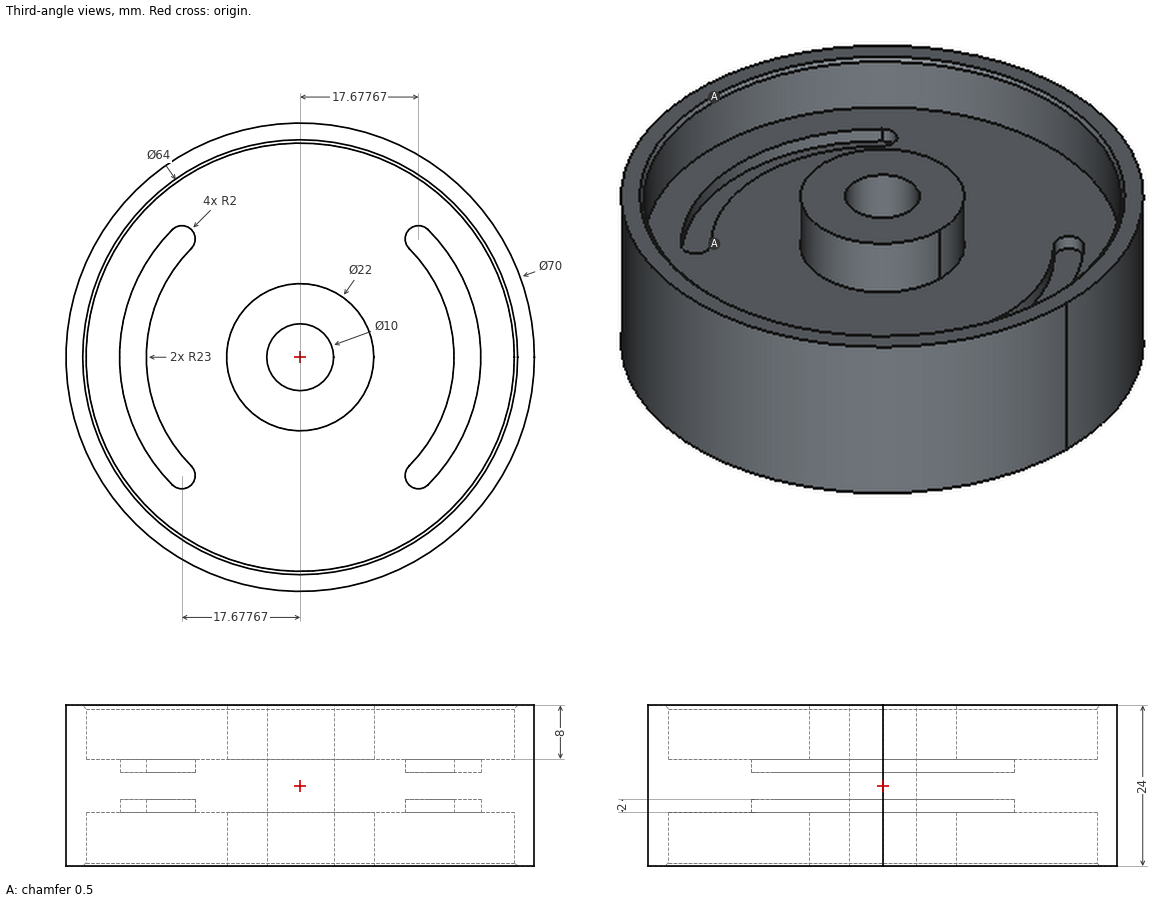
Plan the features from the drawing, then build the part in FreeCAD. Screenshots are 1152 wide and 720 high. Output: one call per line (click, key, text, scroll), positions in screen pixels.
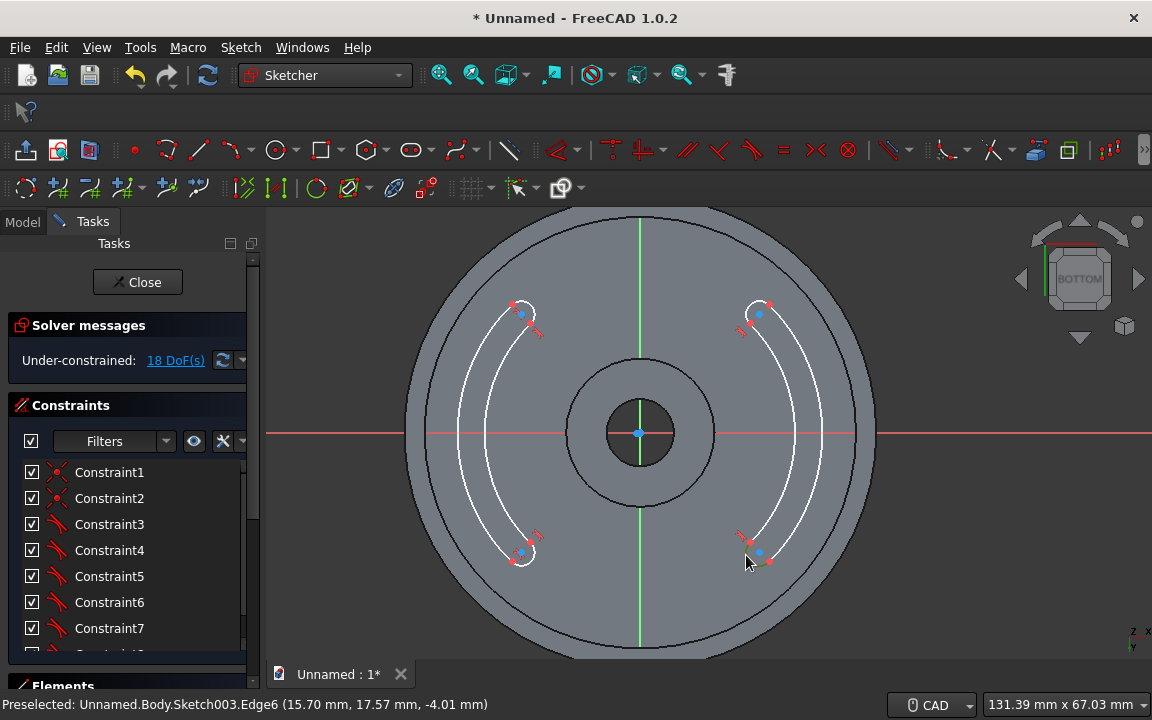
click(813, 490)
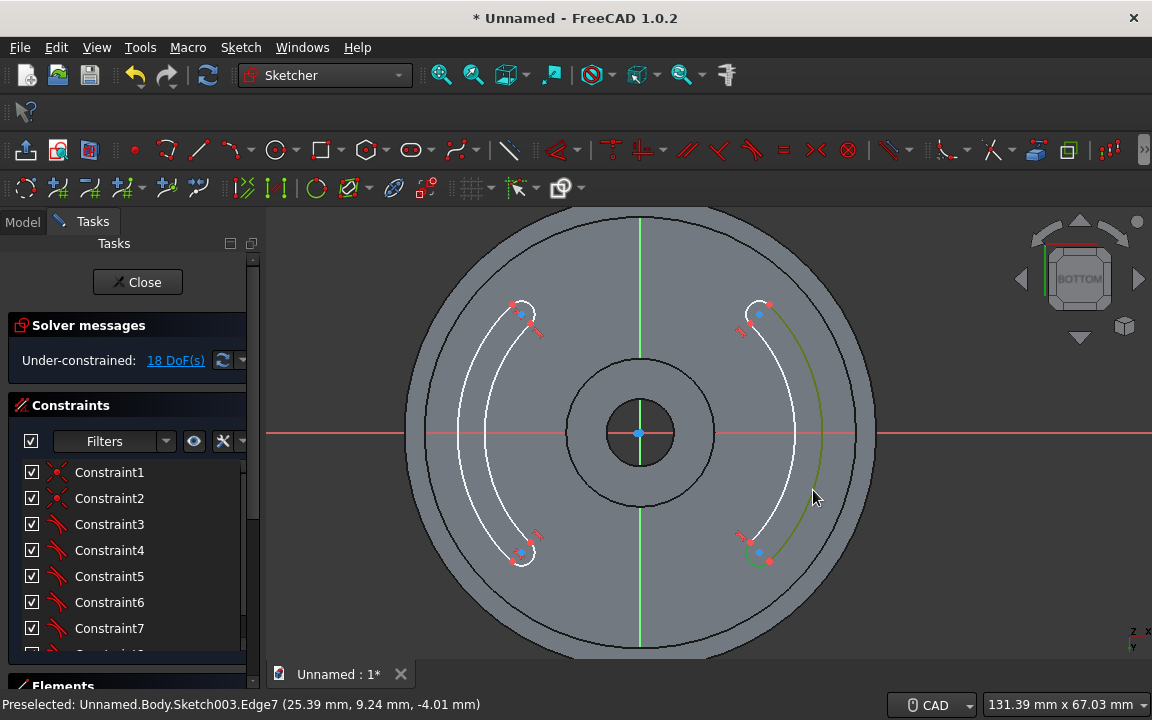
key(t)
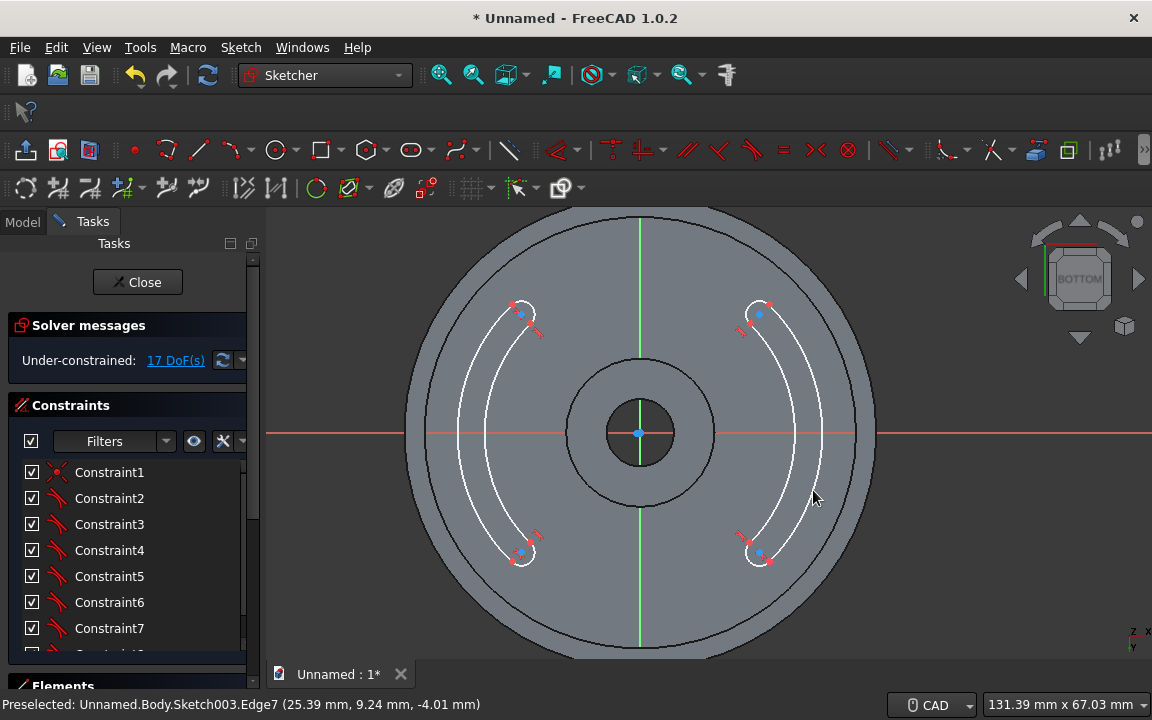
click(813, 490)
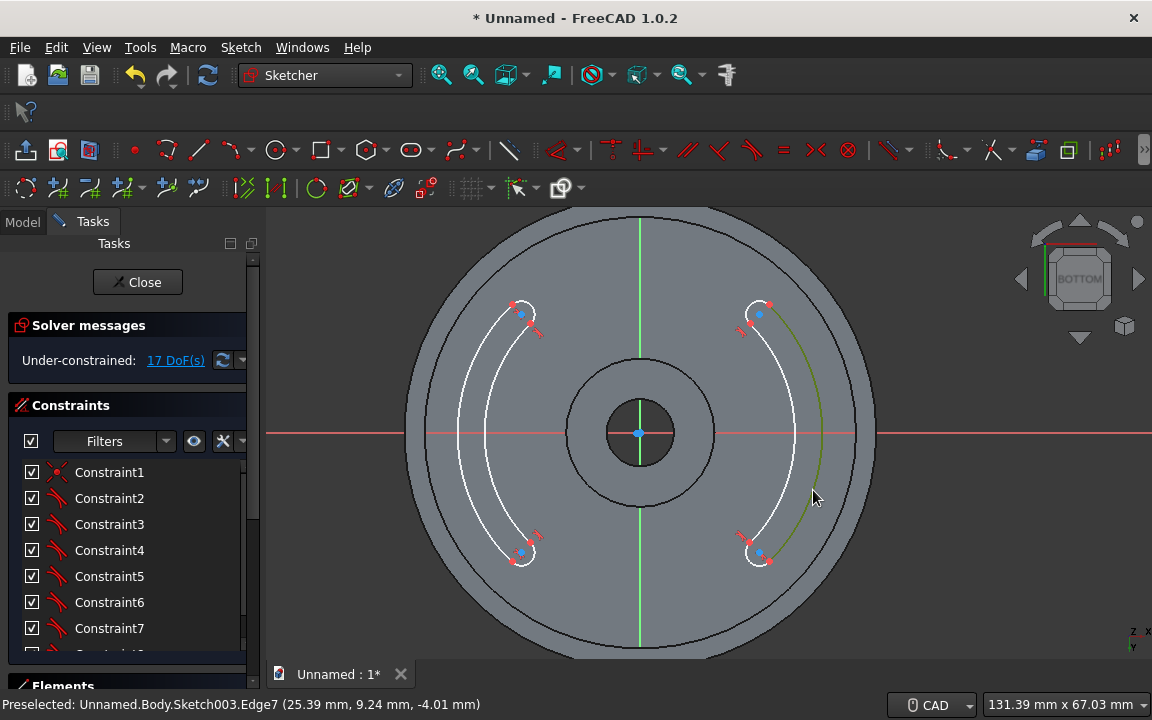
click(757, 301)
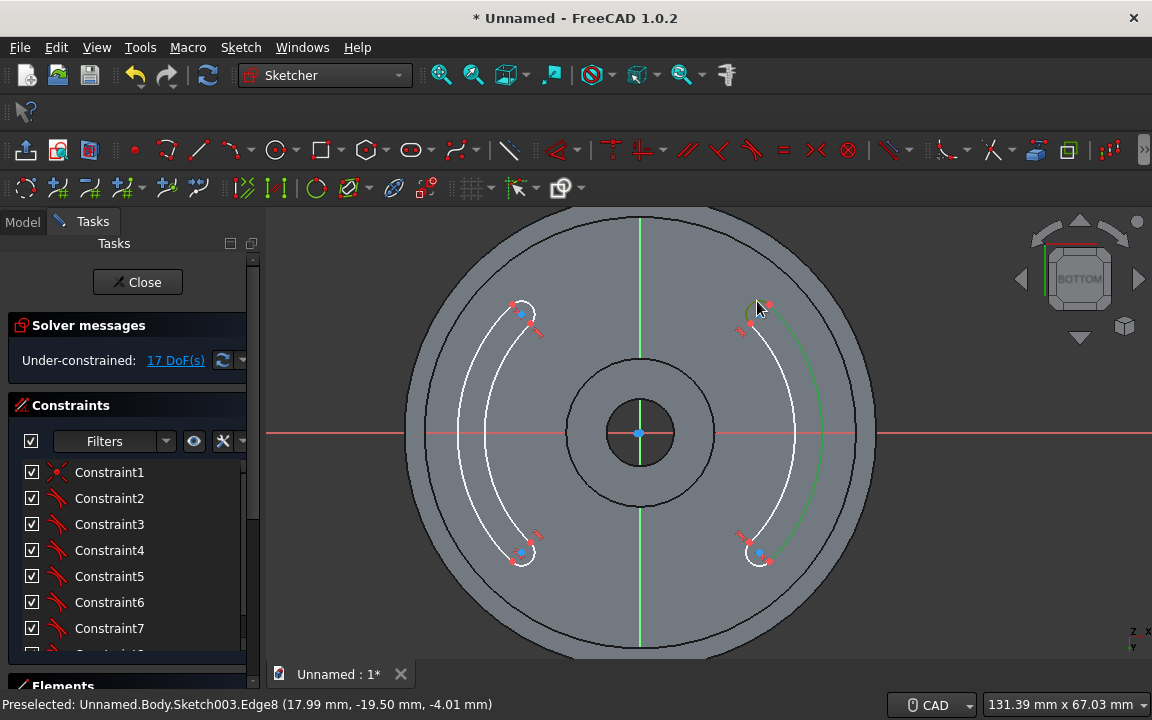
key(t)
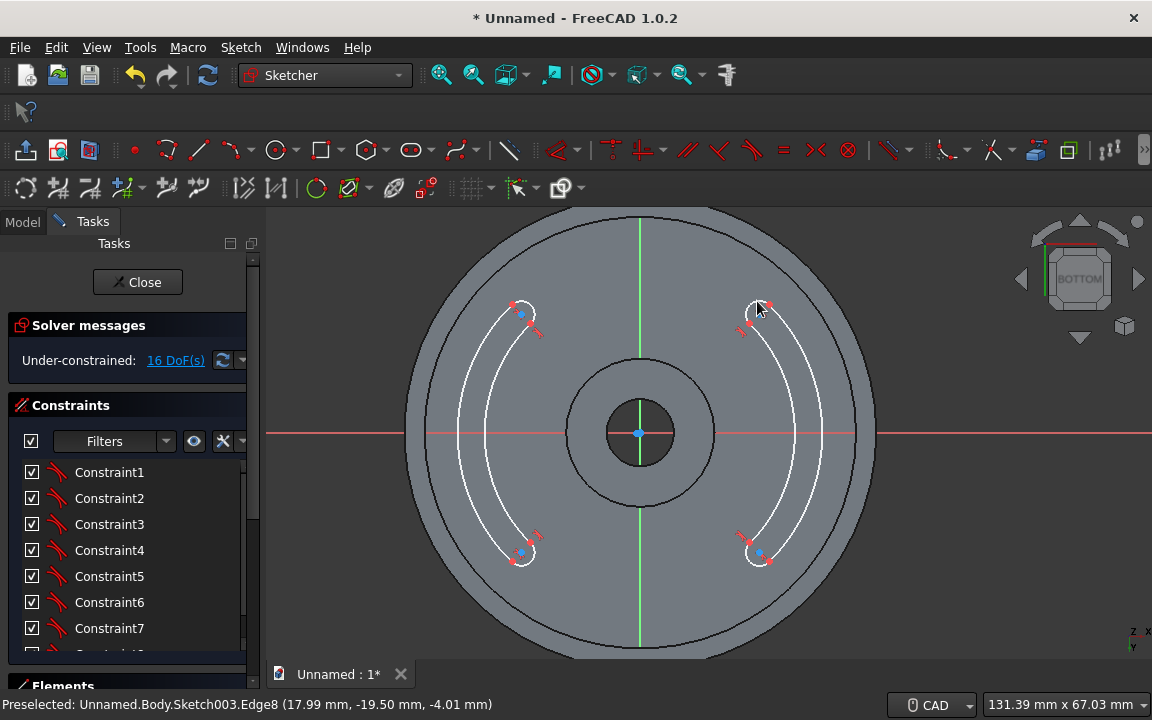
click(492, 386)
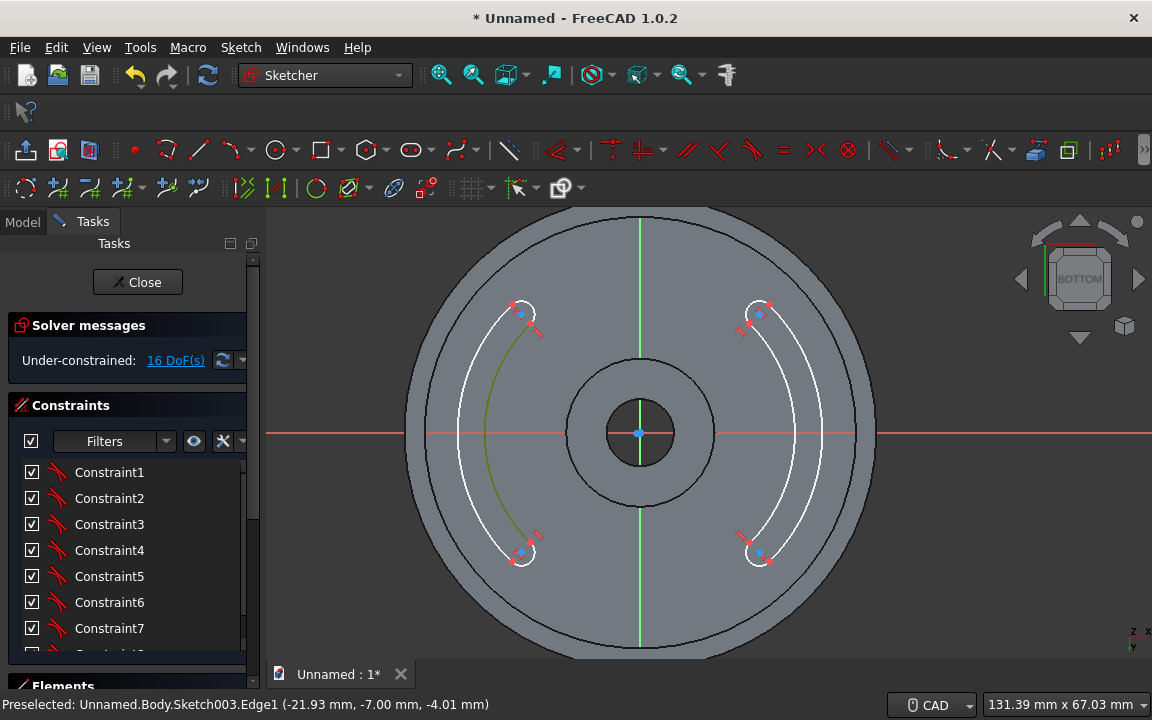
click(467, 377)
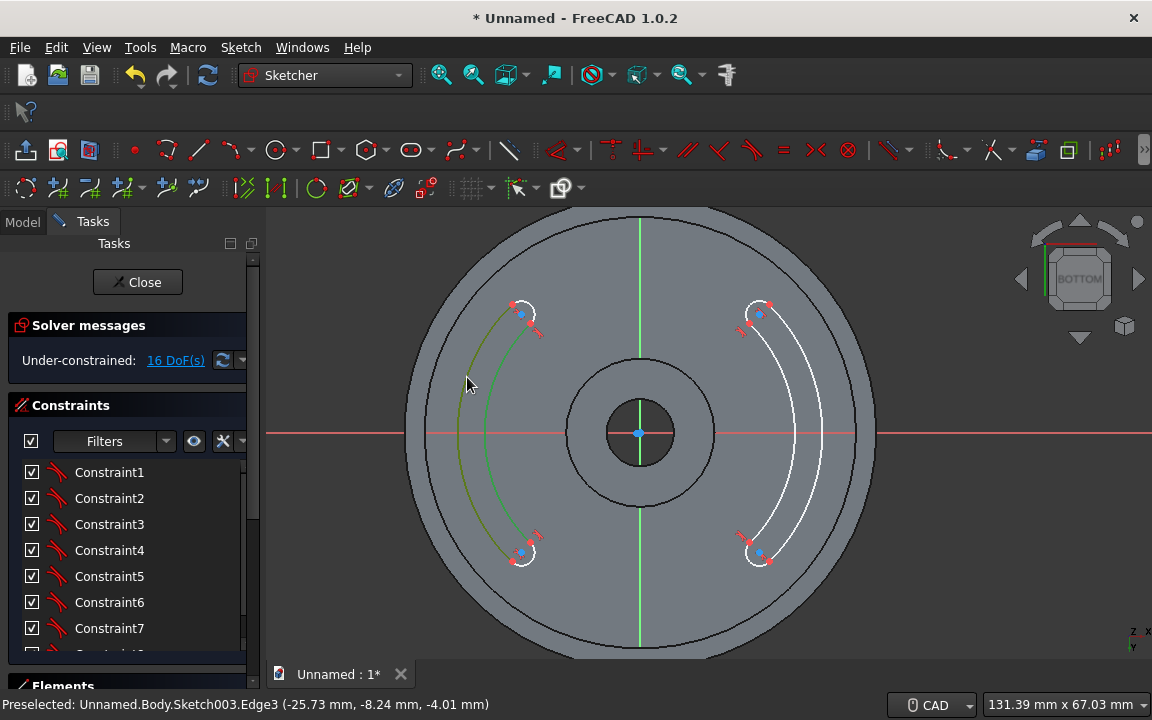
key(c)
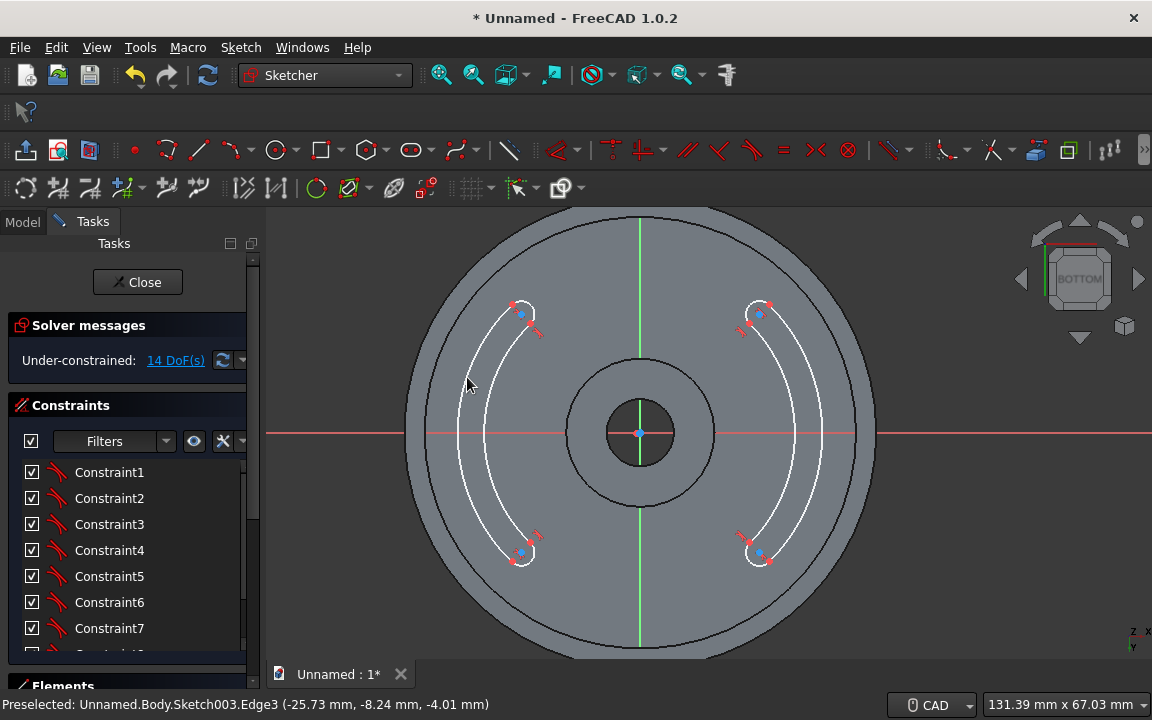
click(492, 385)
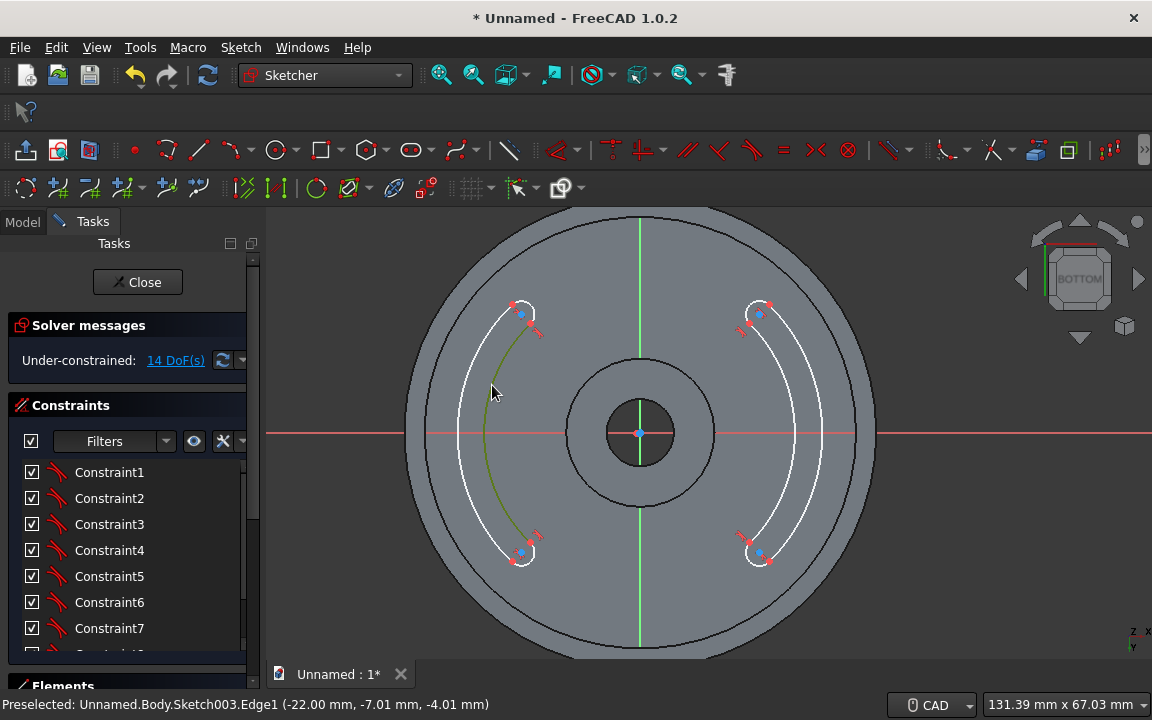
click(787, 481)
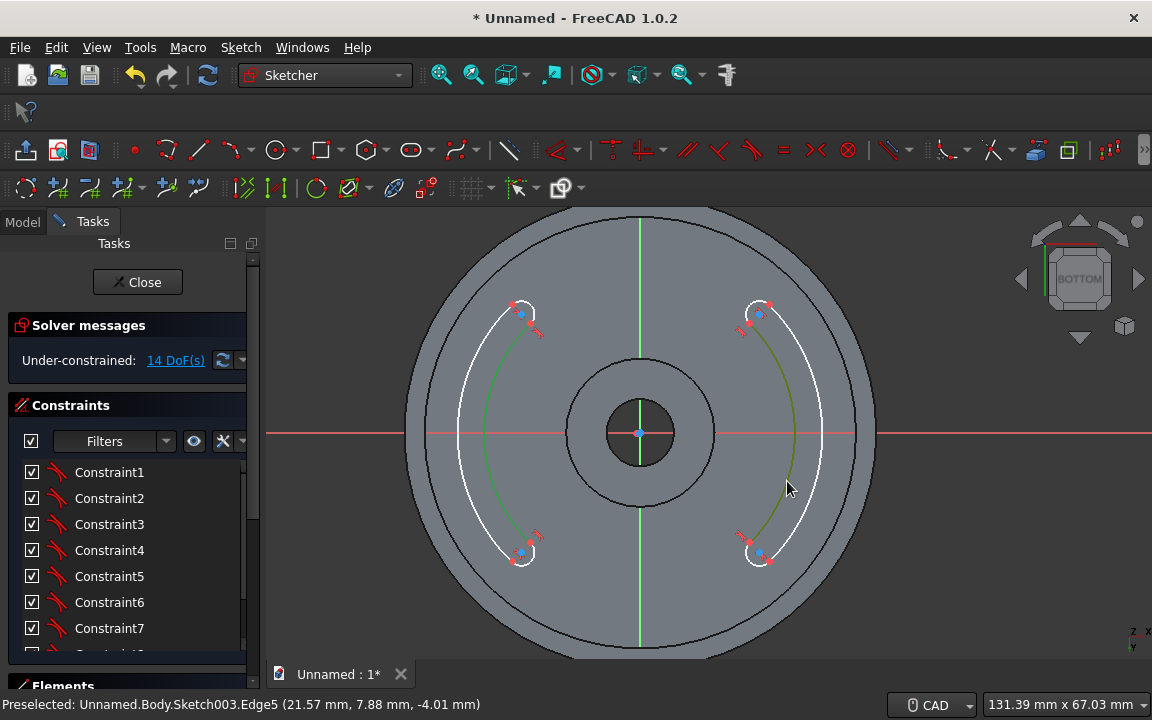
key(c)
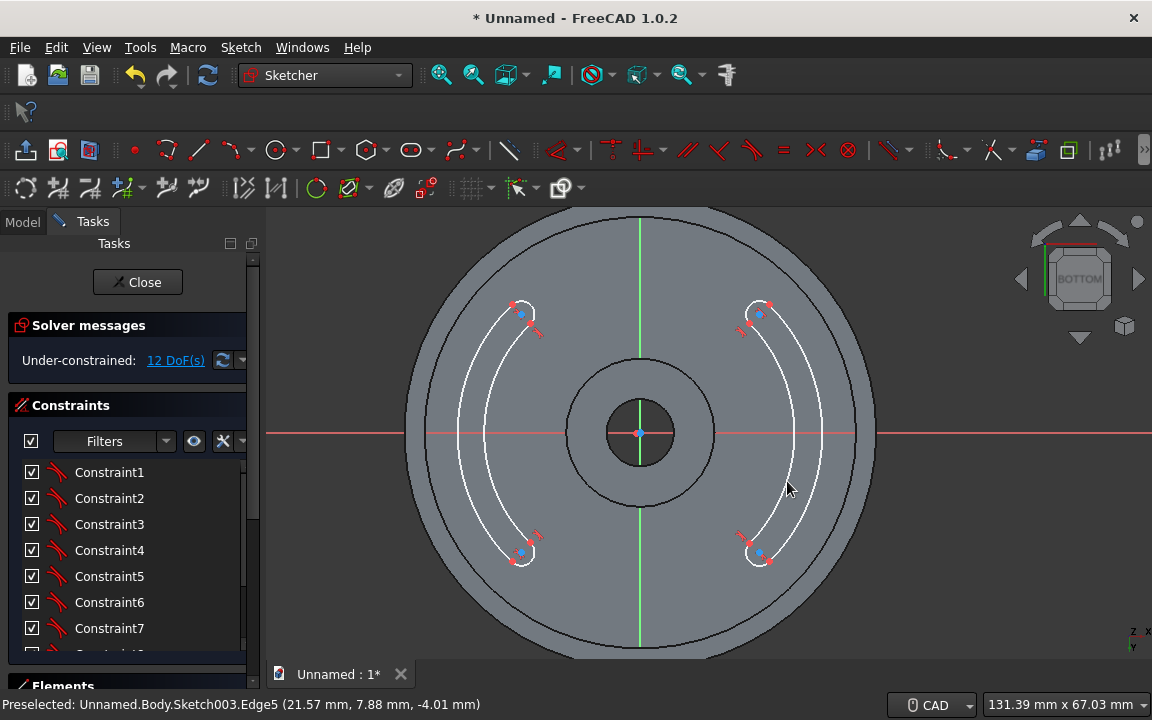
click(492, 385)